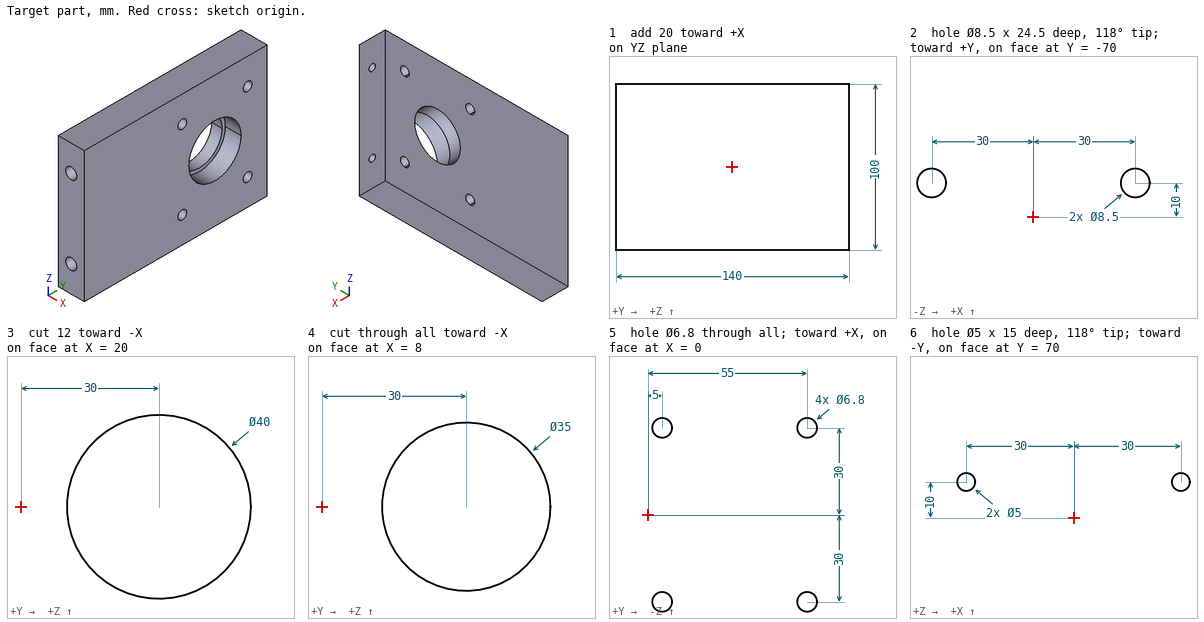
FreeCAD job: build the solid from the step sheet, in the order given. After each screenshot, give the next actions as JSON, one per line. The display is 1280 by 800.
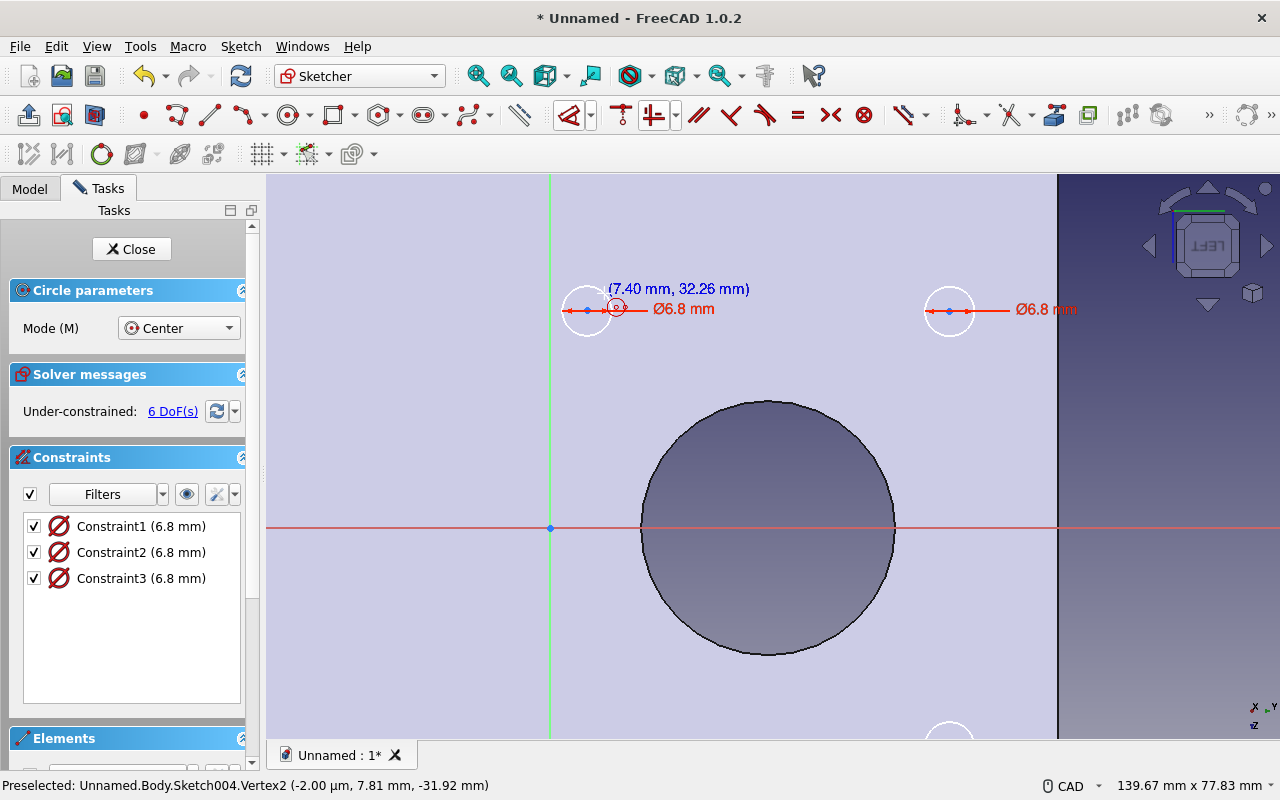
{"action": "scroll", "coordinate": [587, 311], "scroll_direction": "down", "scroll_amount": 2}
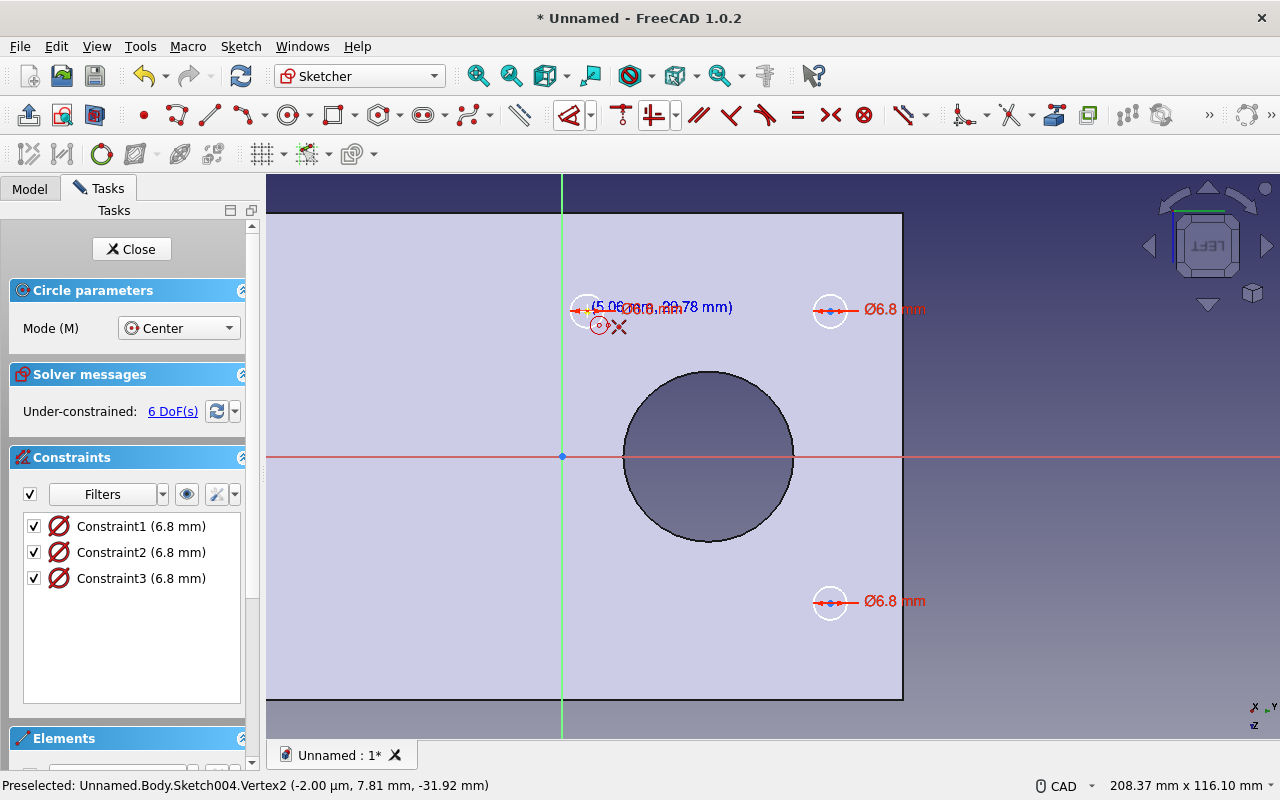
{"action": "scroll", "coordinate": [587, 603], "scroll_direction": "up", "scroll_amount": 2}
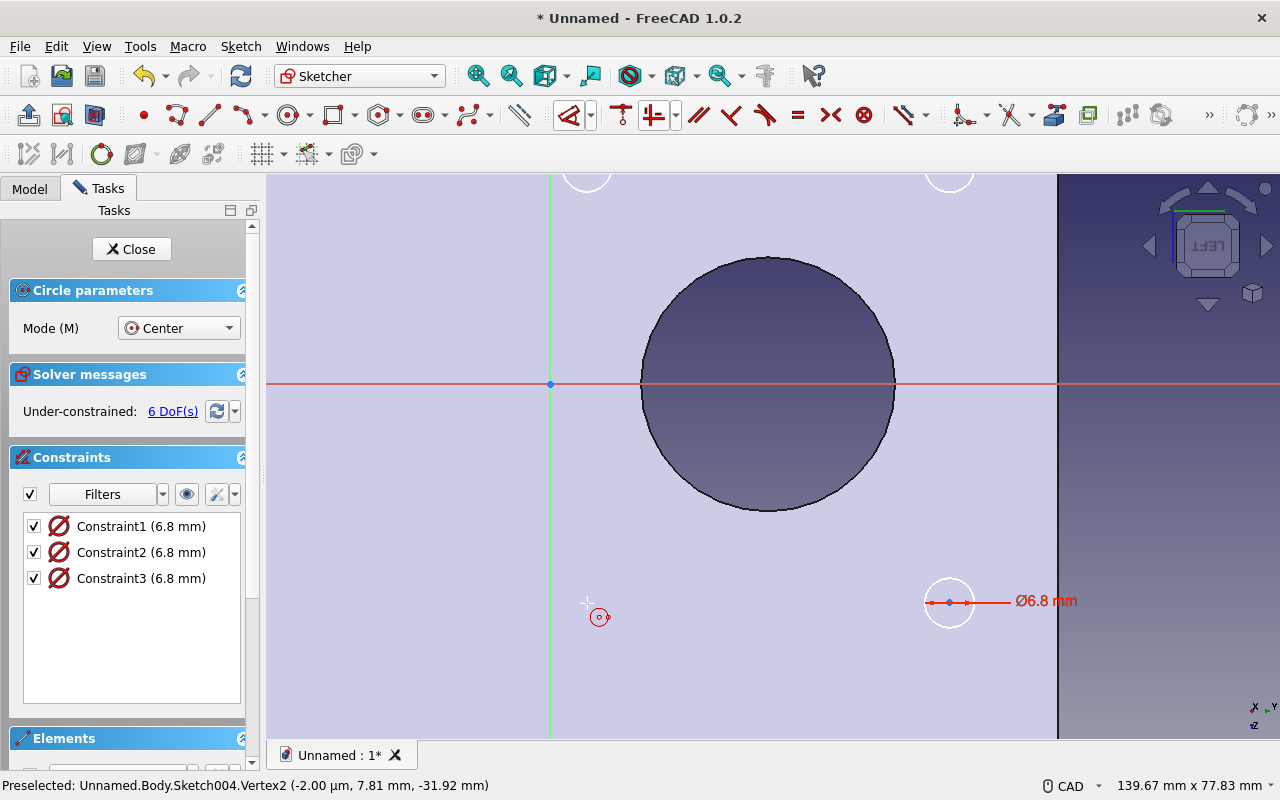
{"action": "left_click", "coordinate": [587, 602]}
{"action": "mouse_move", "coordinate": [604, 585]}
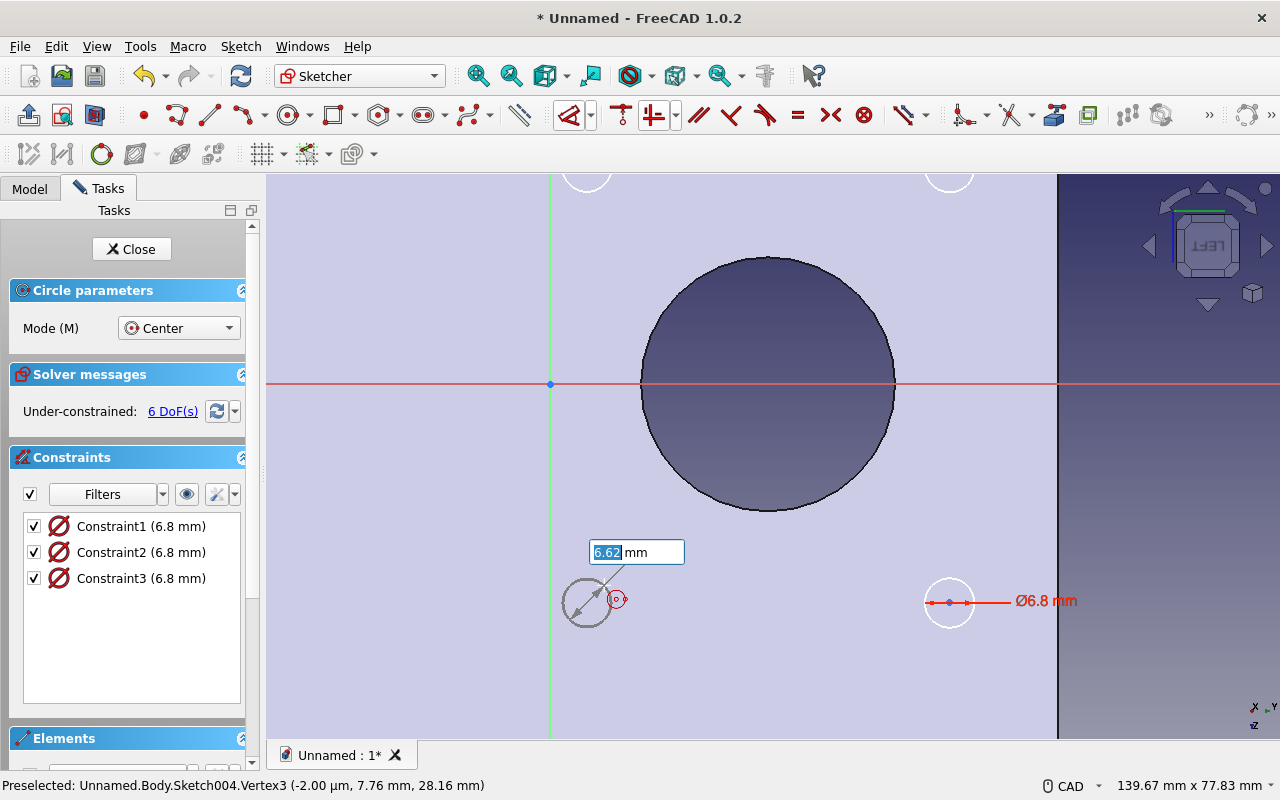
{"action": "type", "text": "6.8"}
{"action": "key", "text": "Return"}
{"action": "key", "text": "Escape"}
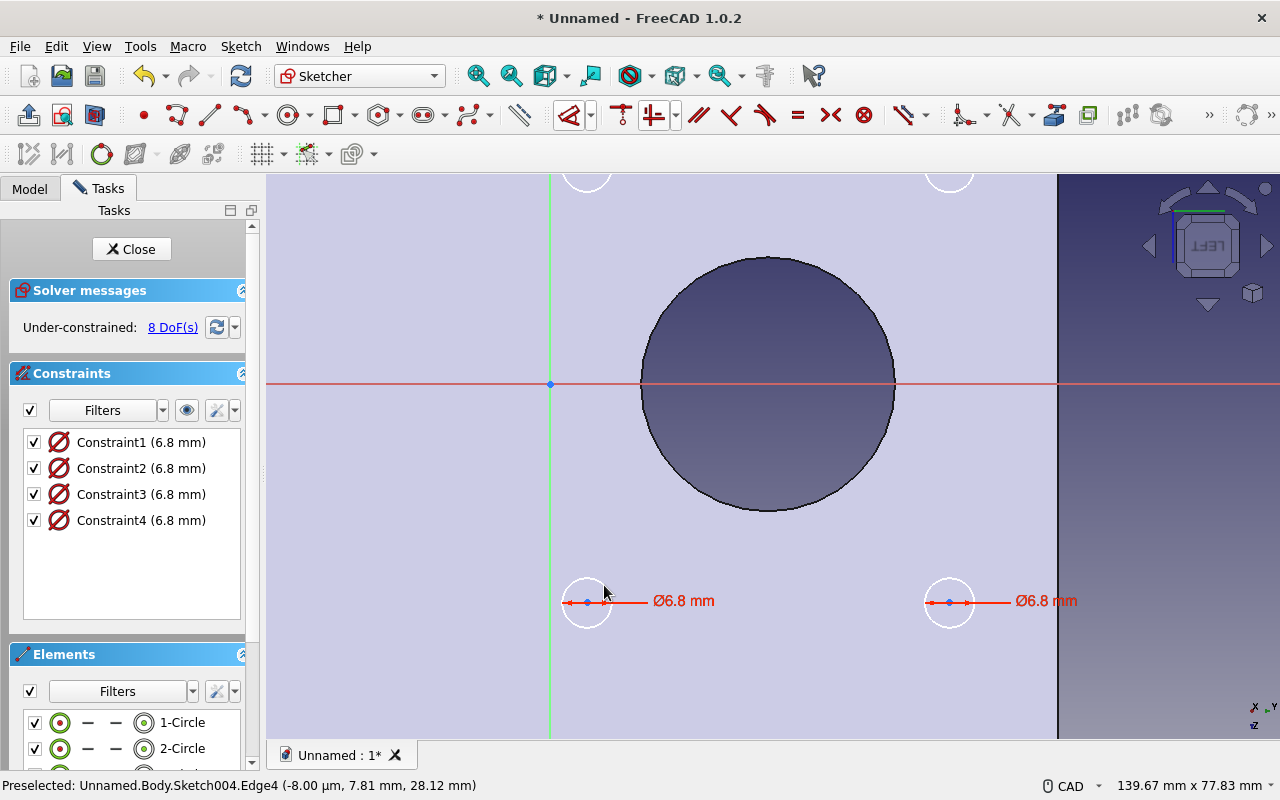
{"action": "scroll", "coordinate": [587, 603], "scroll_direction": "down", "scroll_amount": 2}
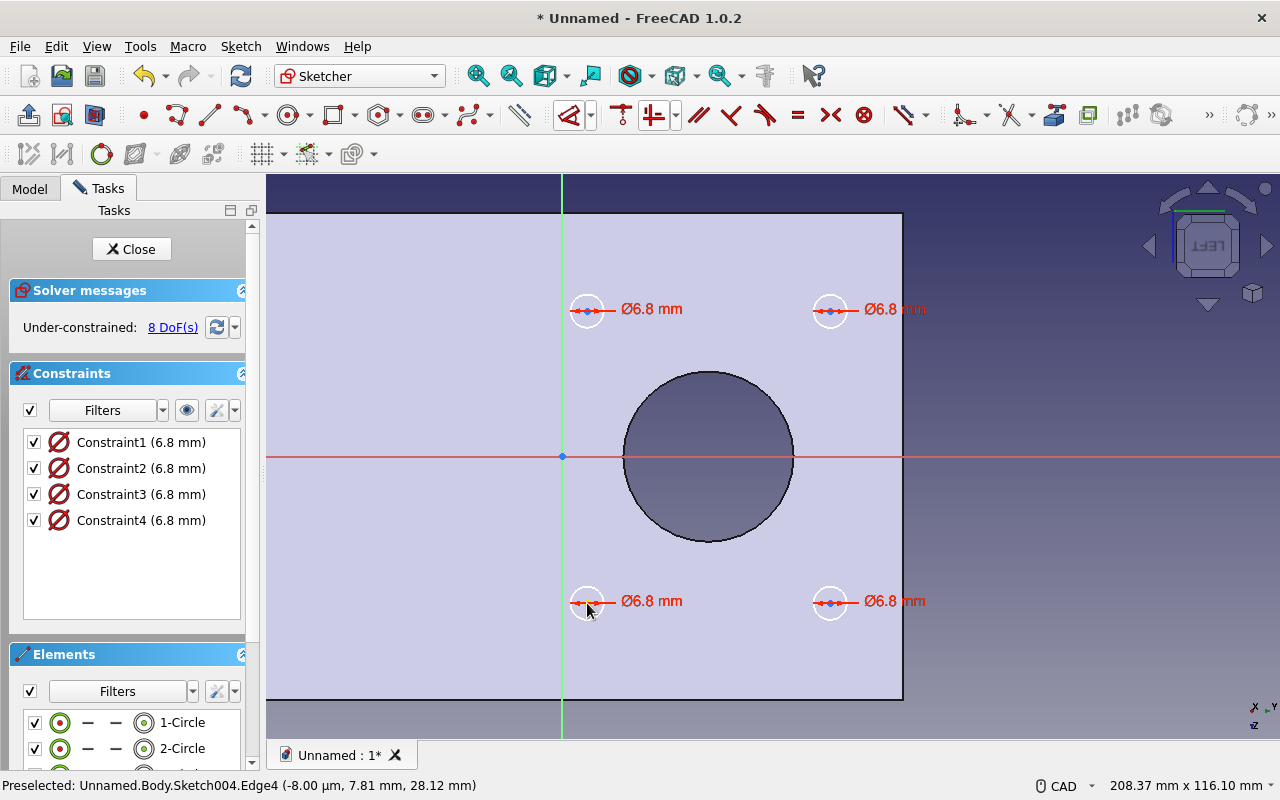
{"action": "left_click", "coordinate": [830, 311]}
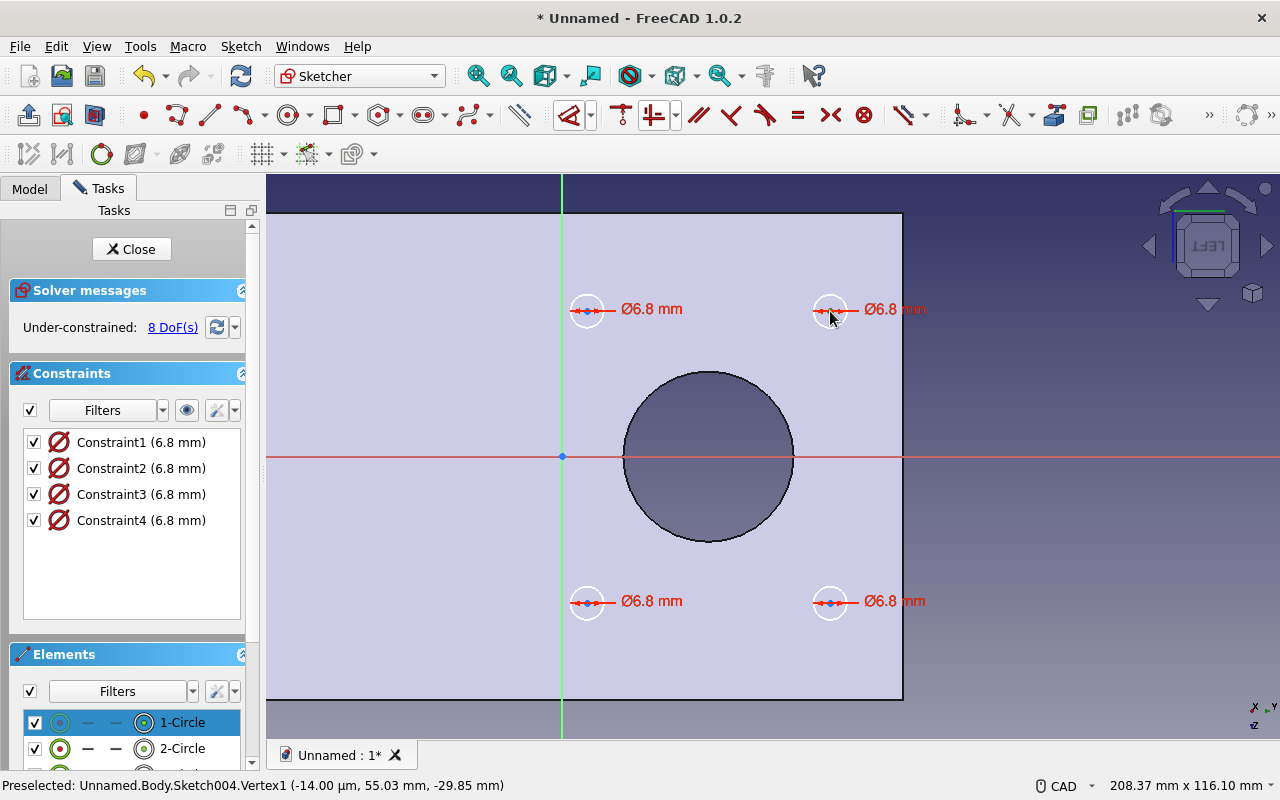
{"action": "left_click", "coordinate": [830, 603]}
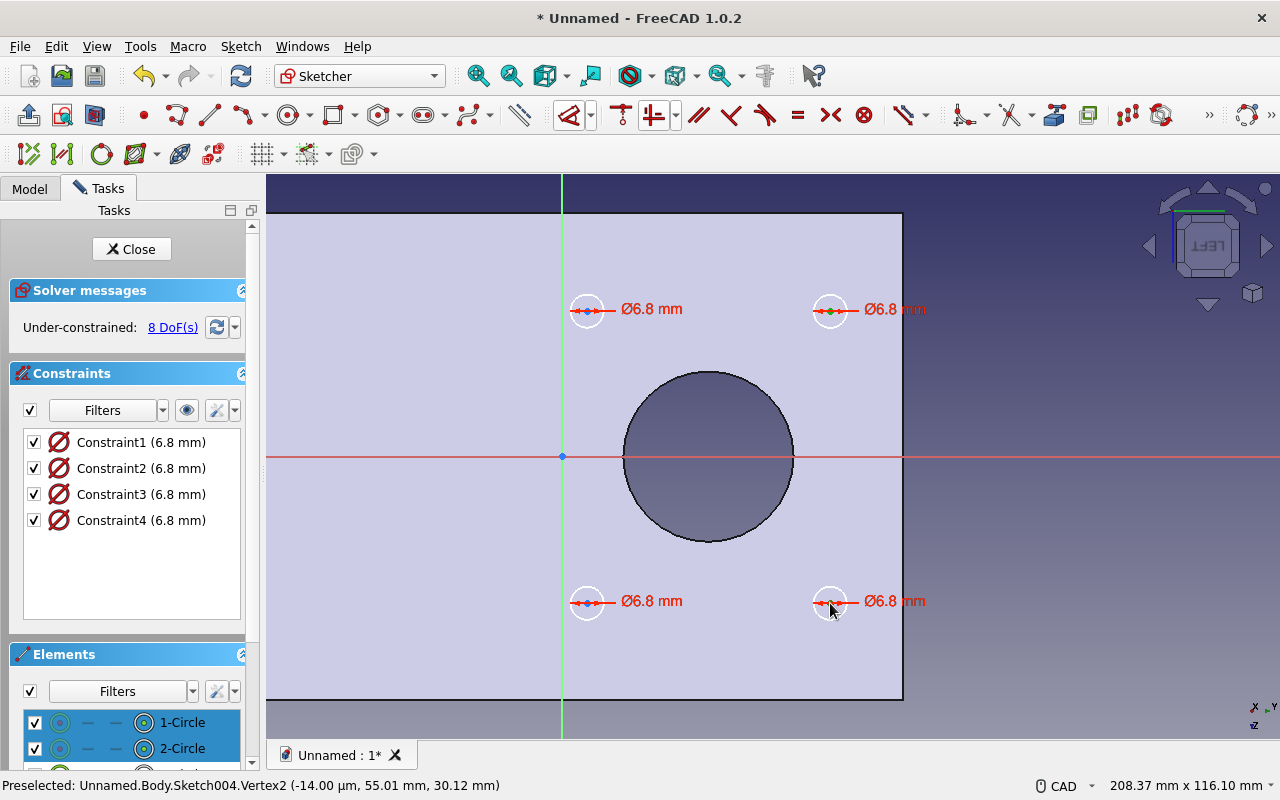
{"action": "key", "text": "v"}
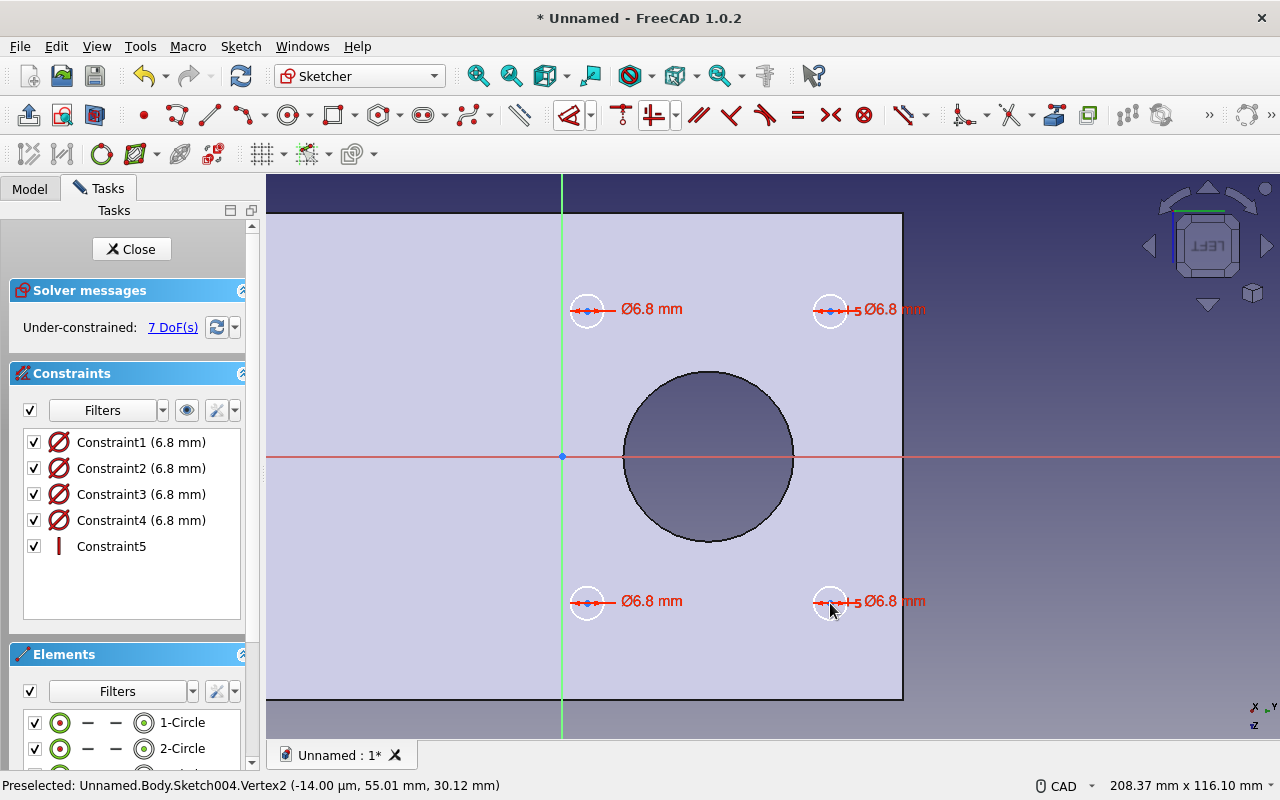
{"action": "left_click", "coordinate": [830, 311]}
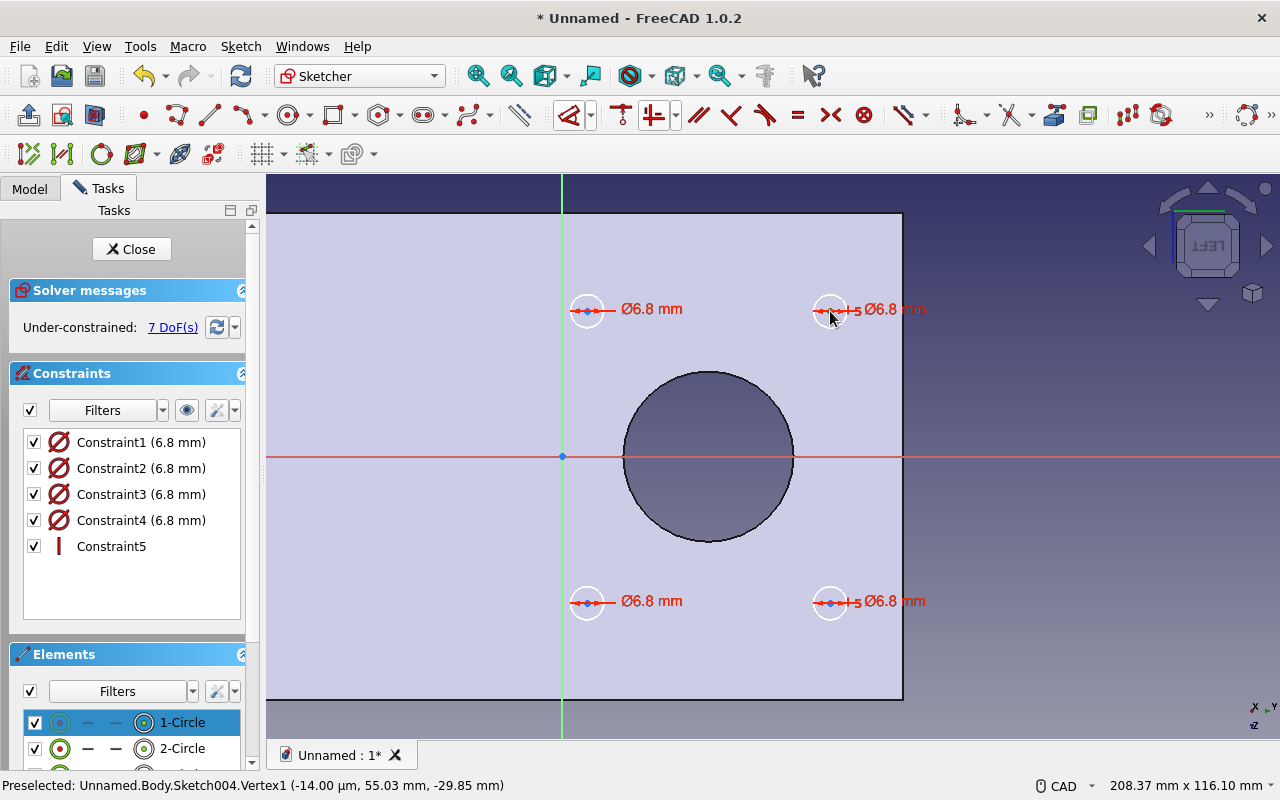
{"action": "left_click", "coordinate": [587, 311]}